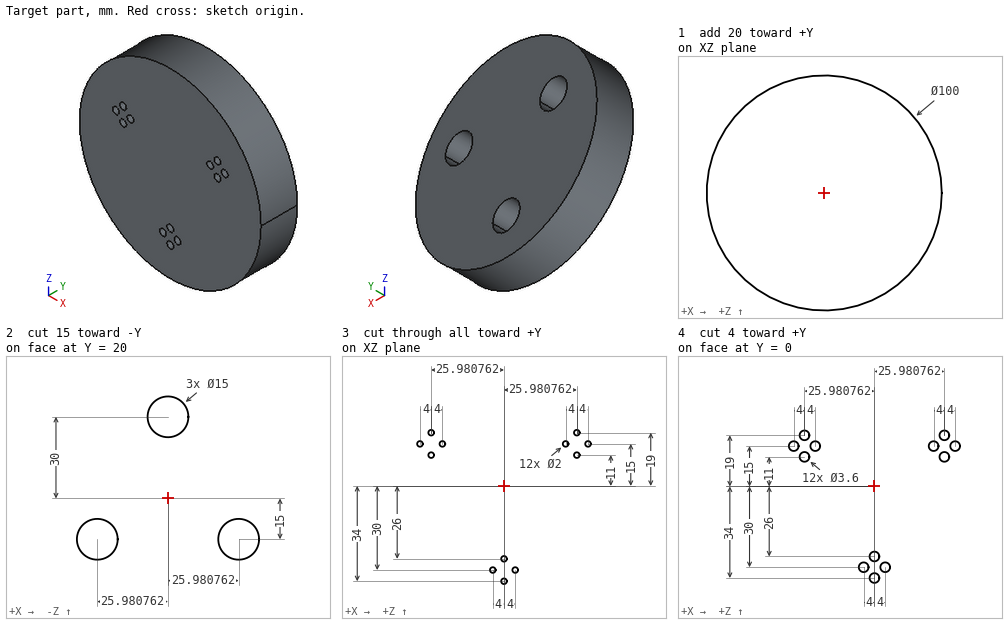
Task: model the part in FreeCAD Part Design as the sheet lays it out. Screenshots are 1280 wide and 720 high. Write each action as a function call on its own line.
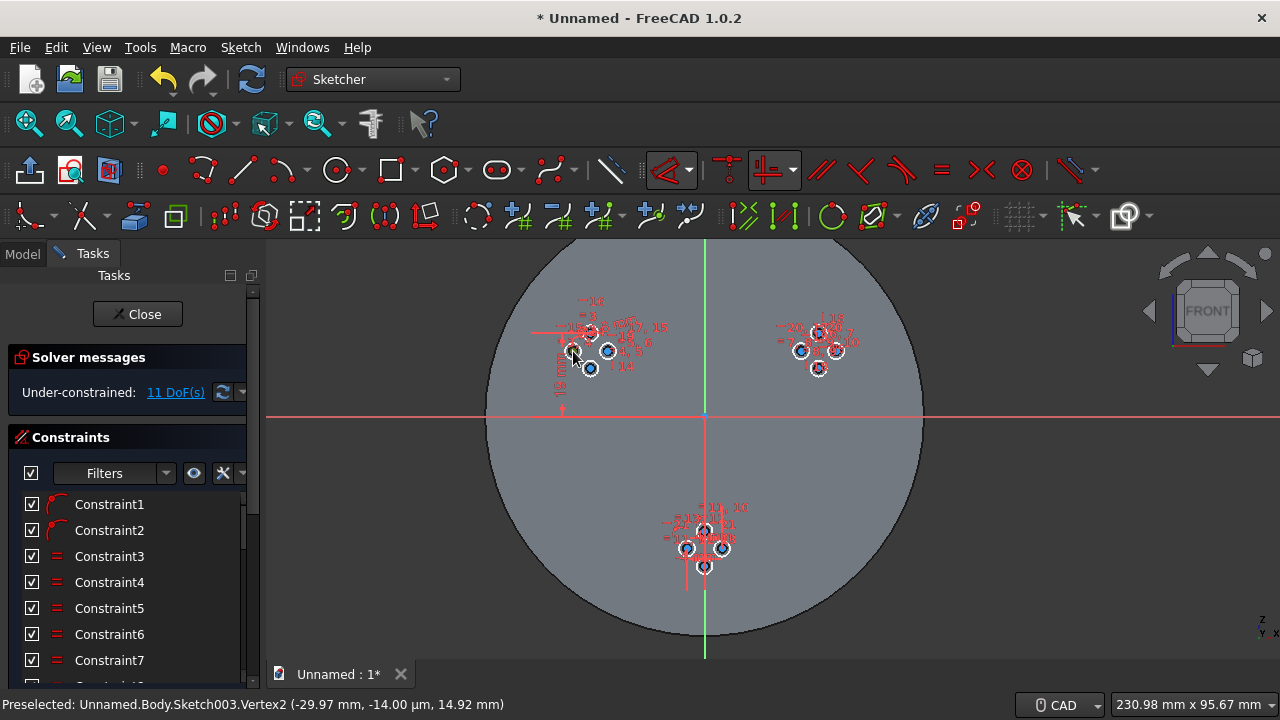
click(692, 170)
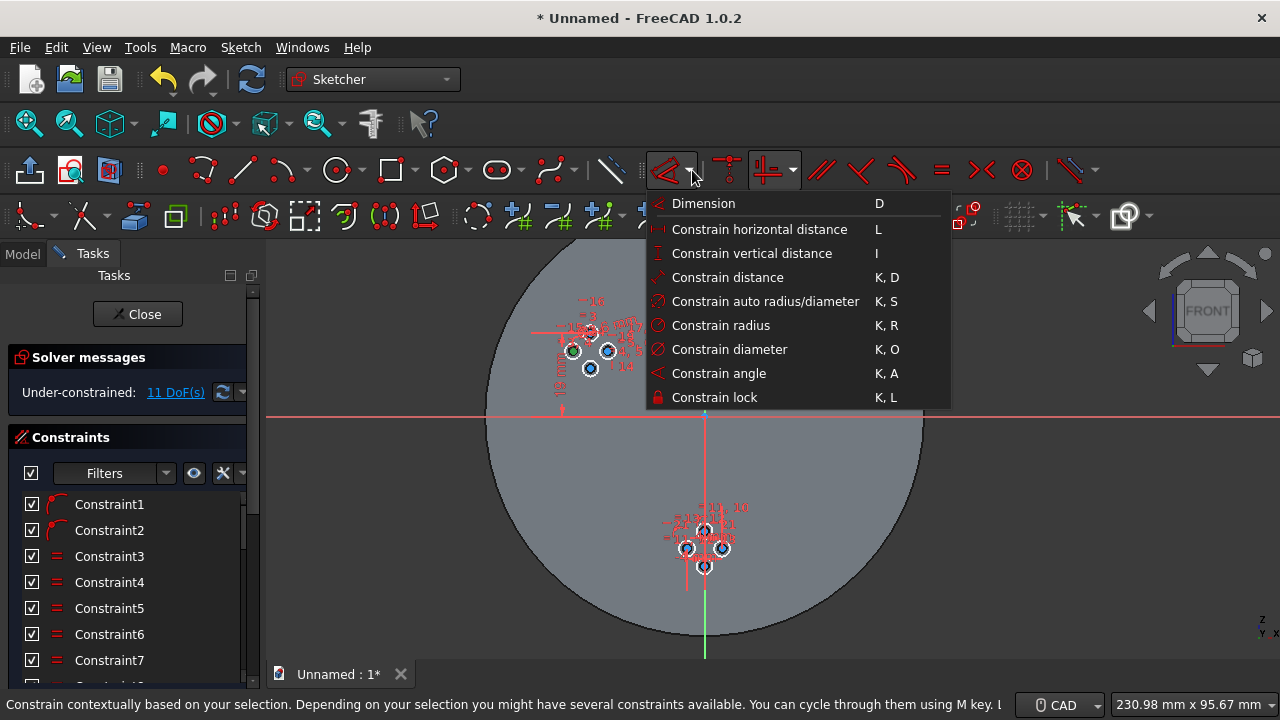
click(799, 253)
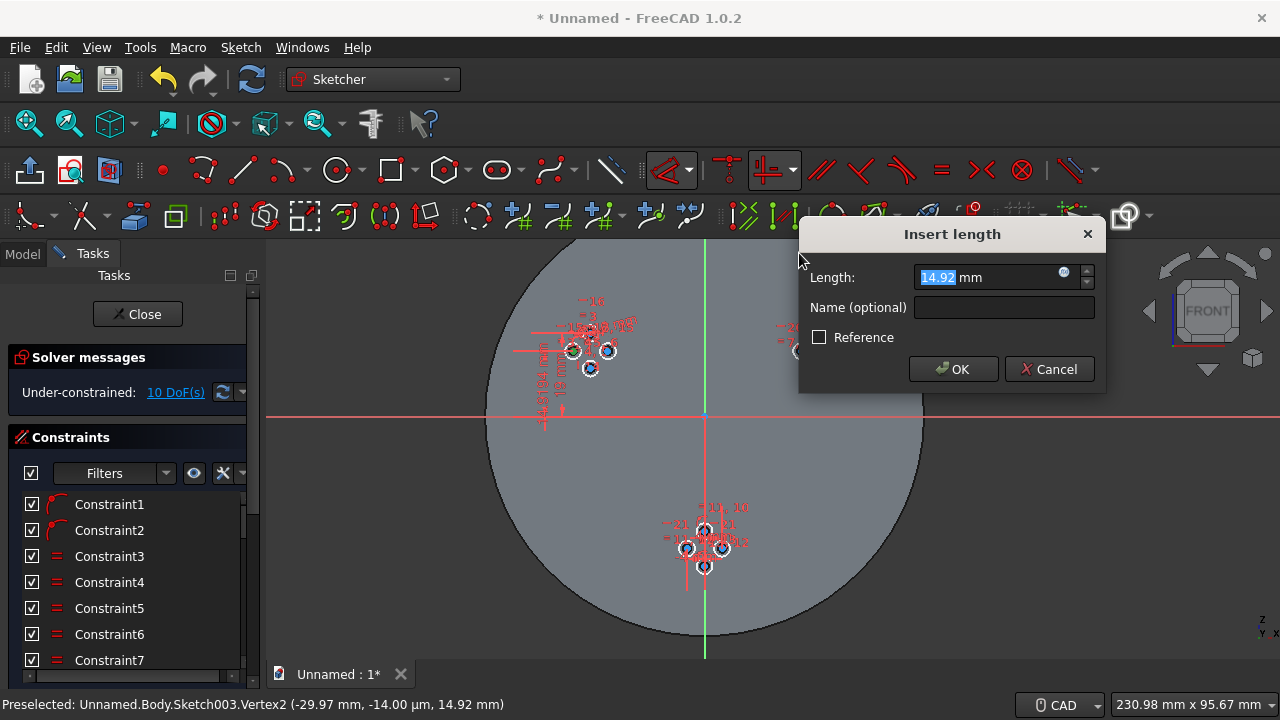
text(15)
key(Return)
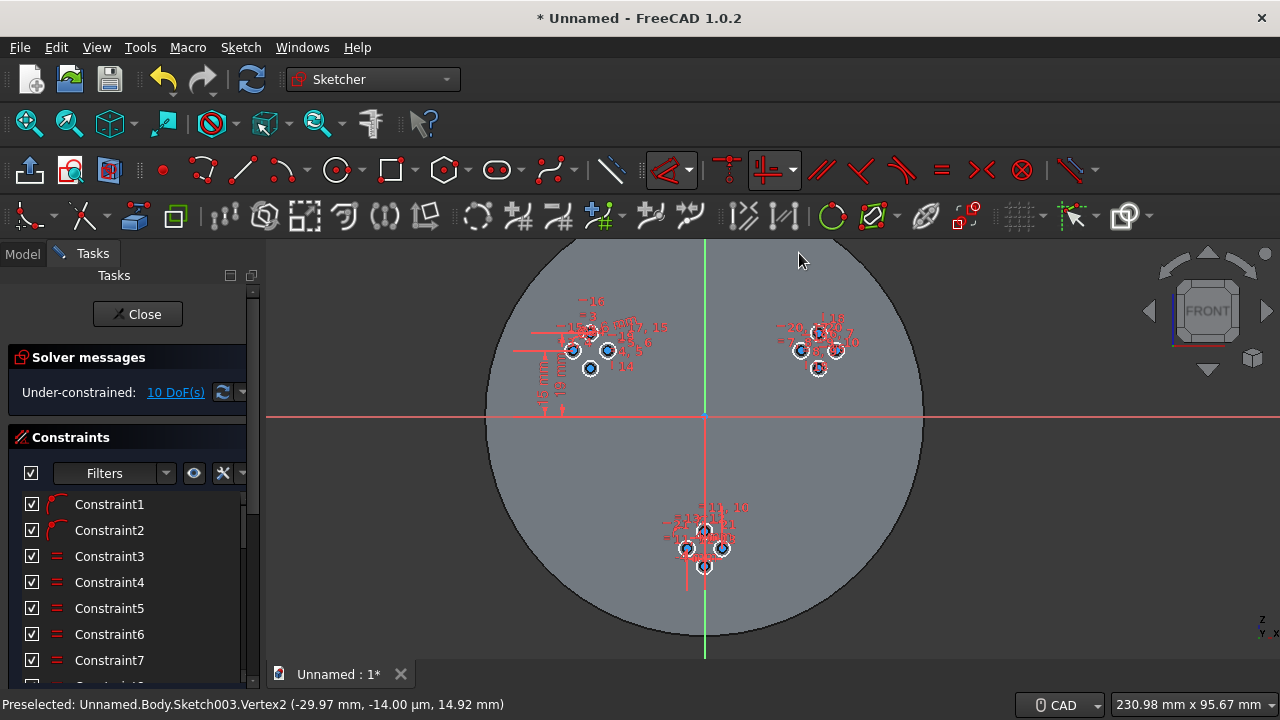
click(590, 369)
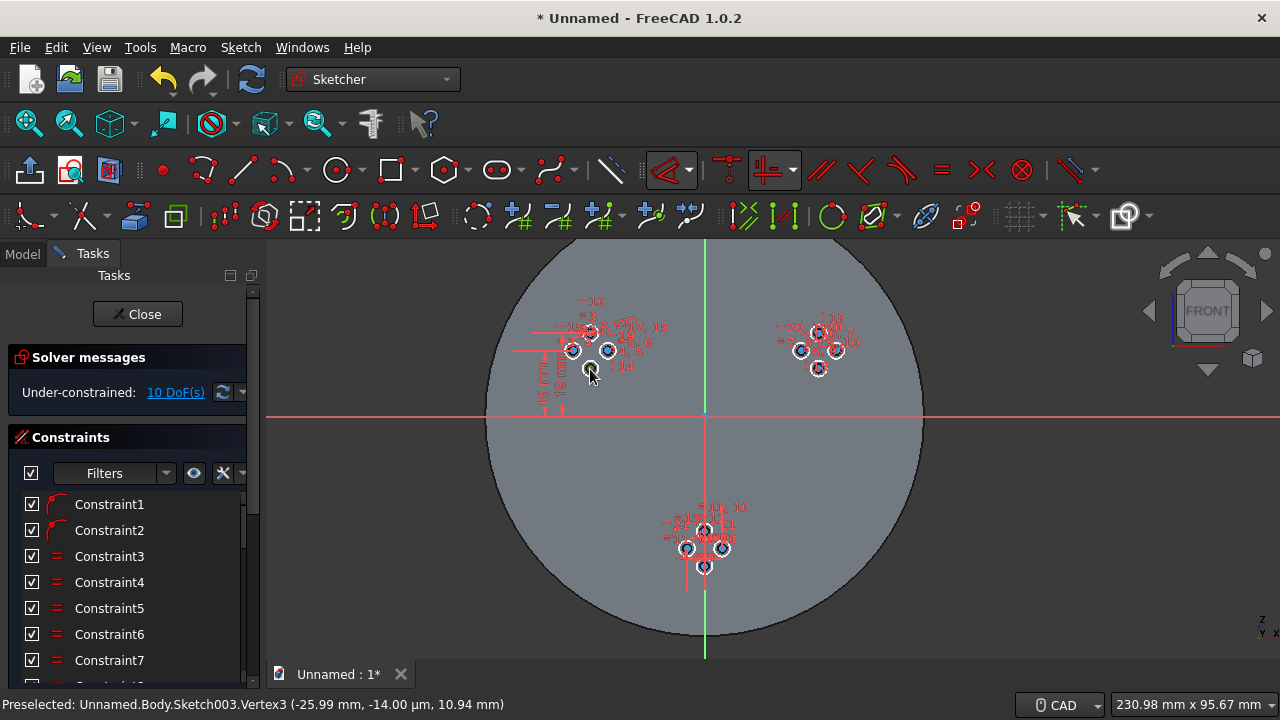
click(692, 170)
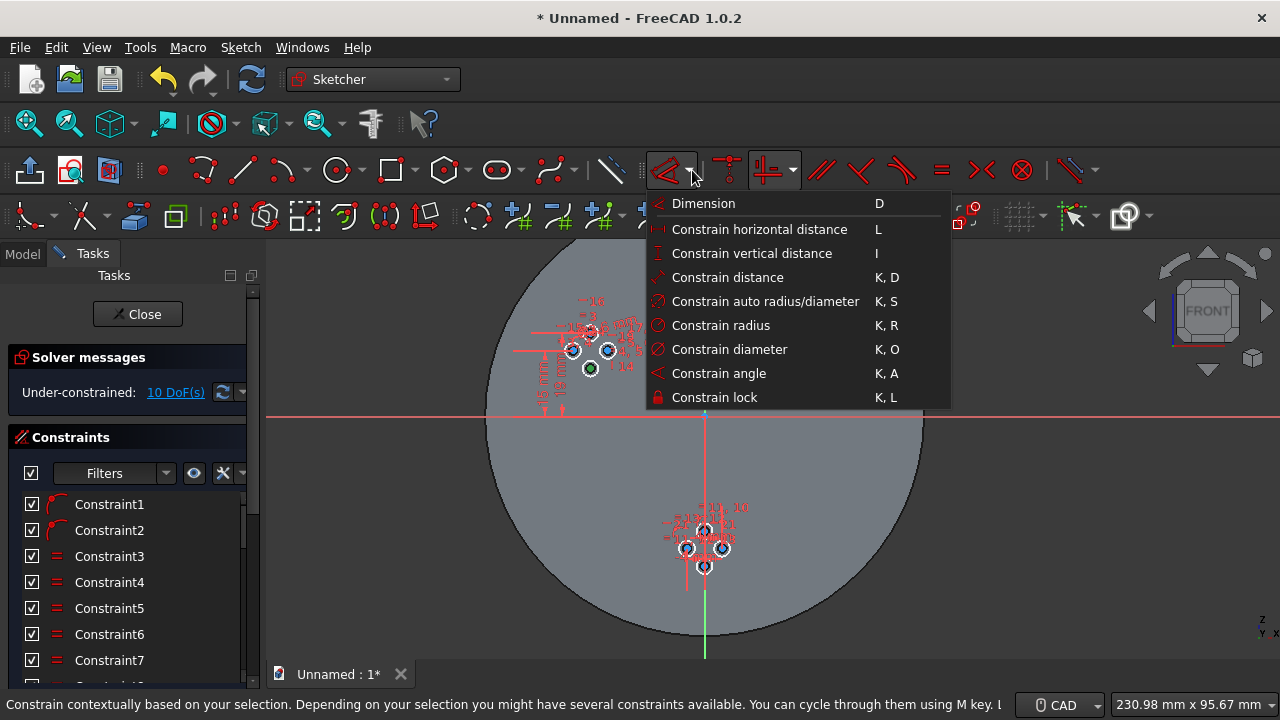
click(799, 253)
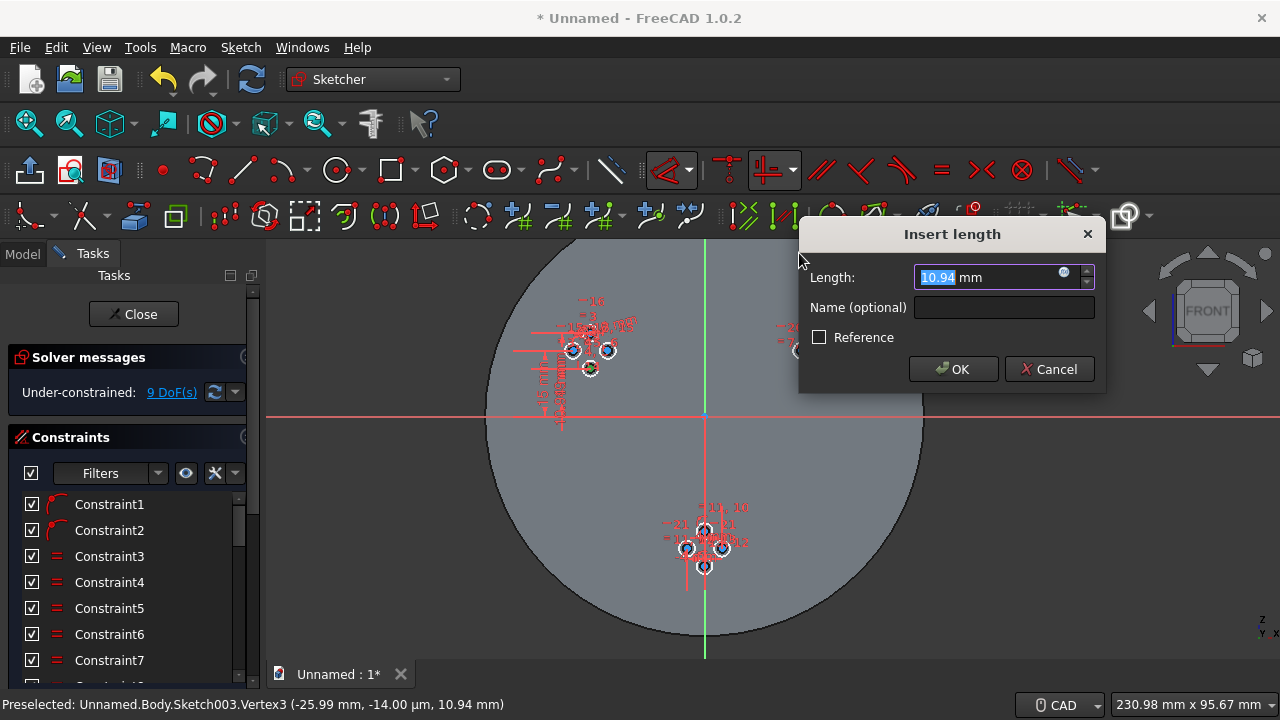
text(11)
key(Return)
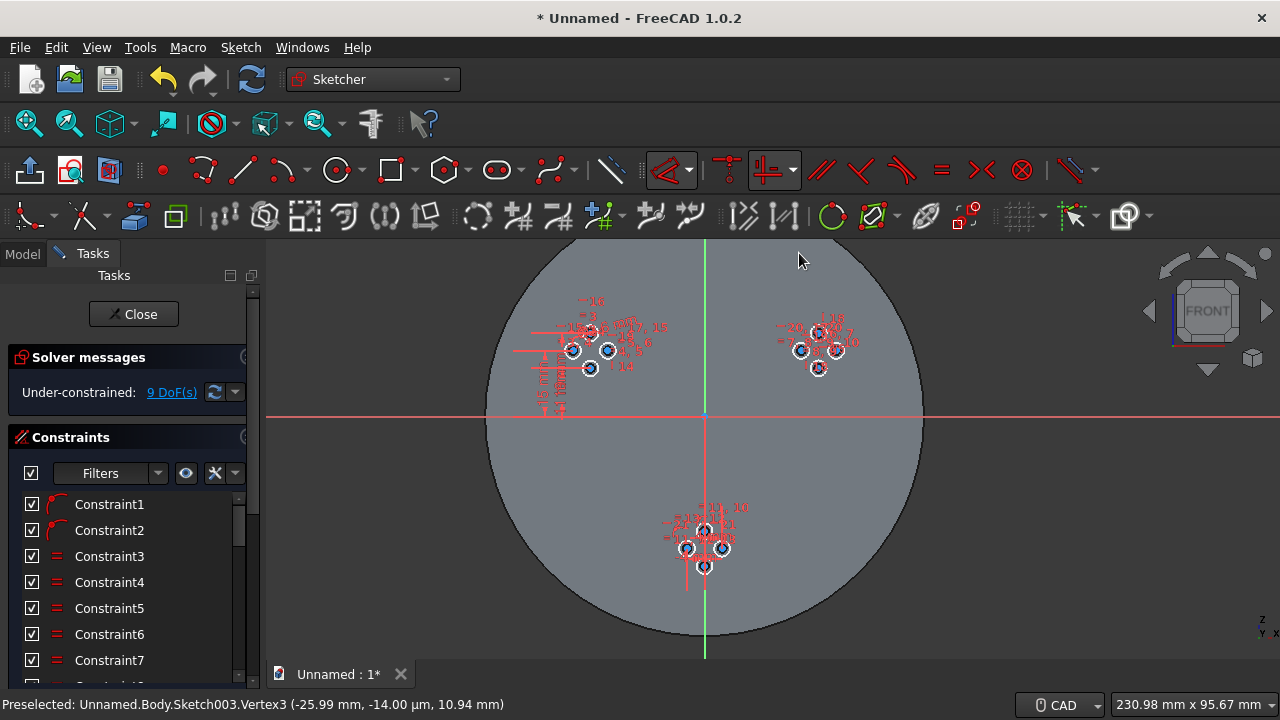
click(705, 531)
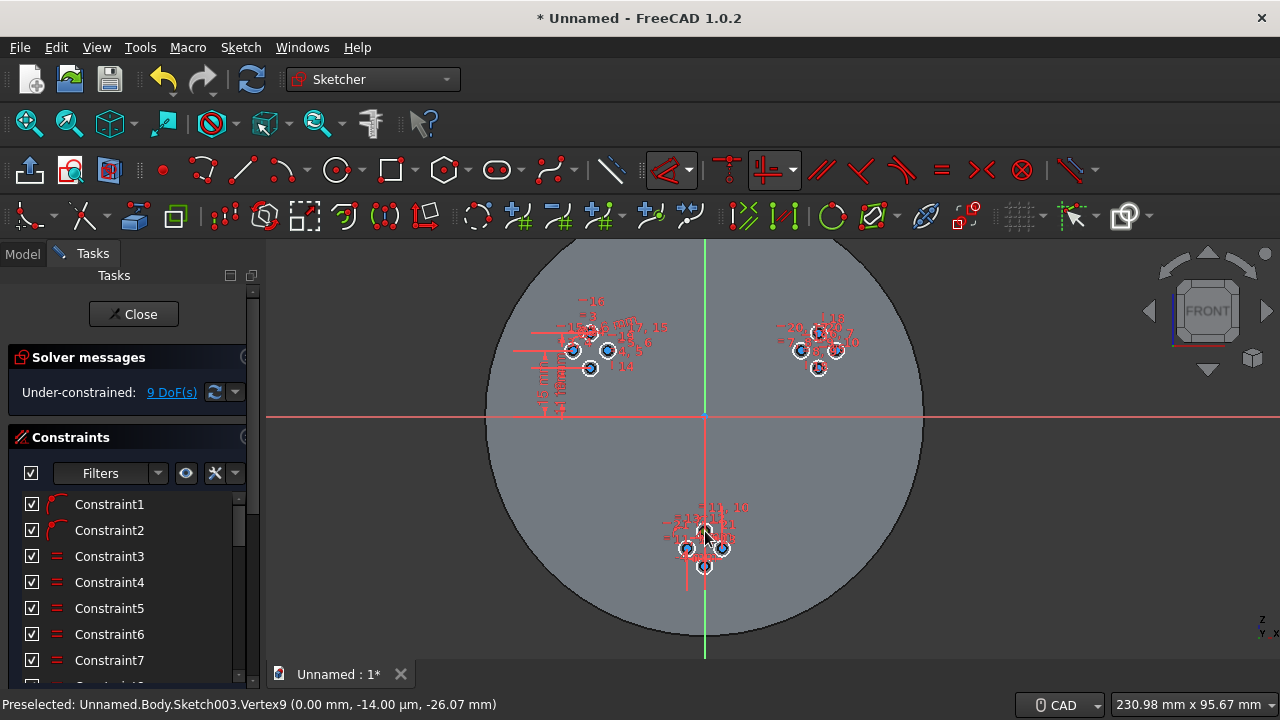
key(i)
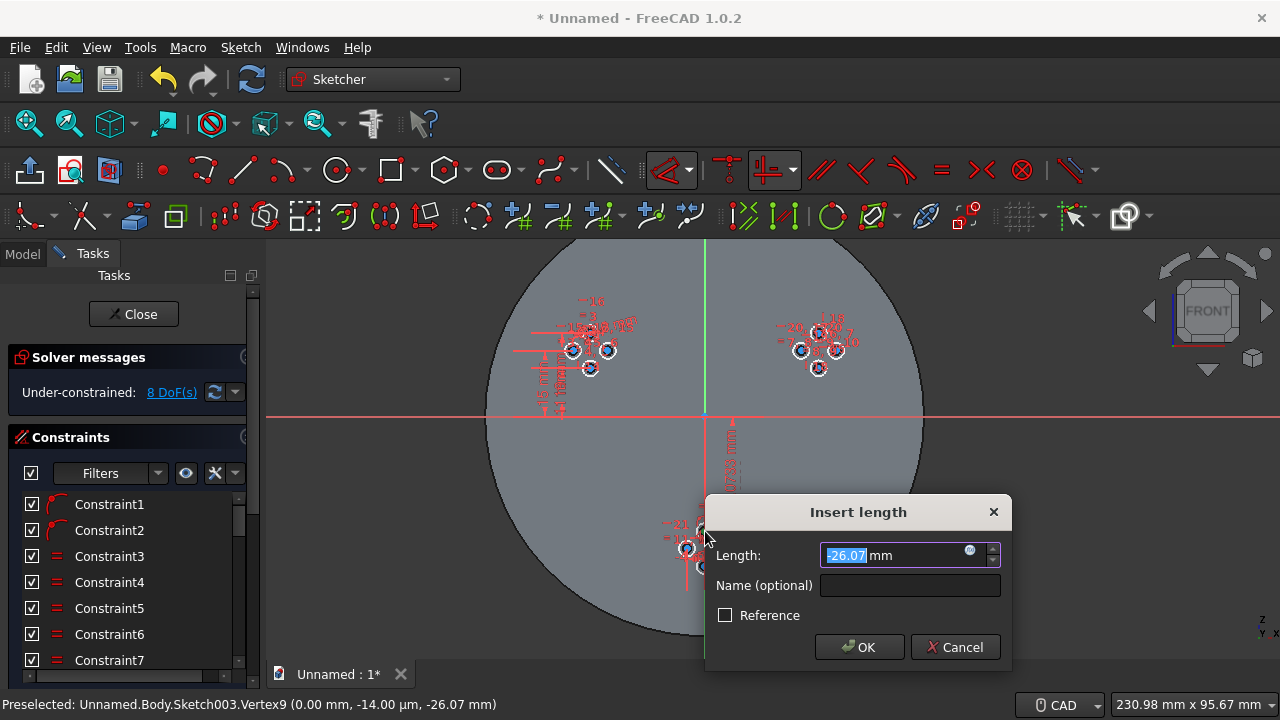
text(-26)
key(Return)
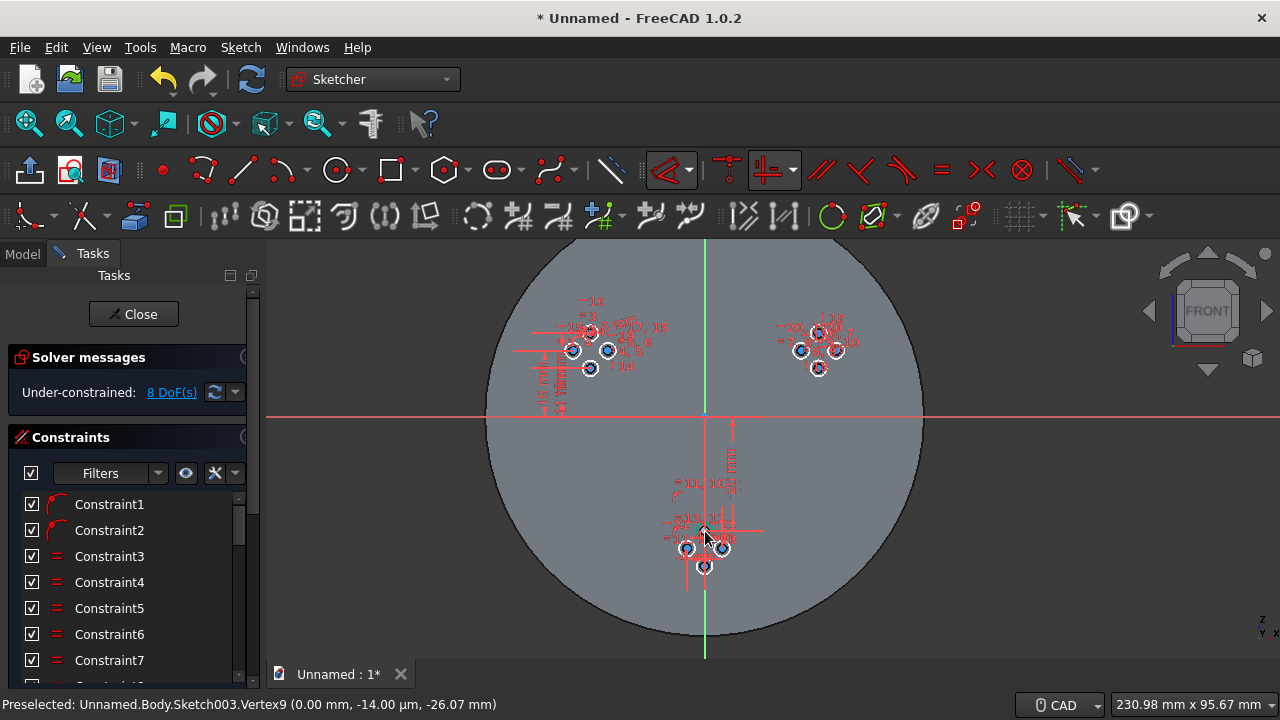
click(687, 549)